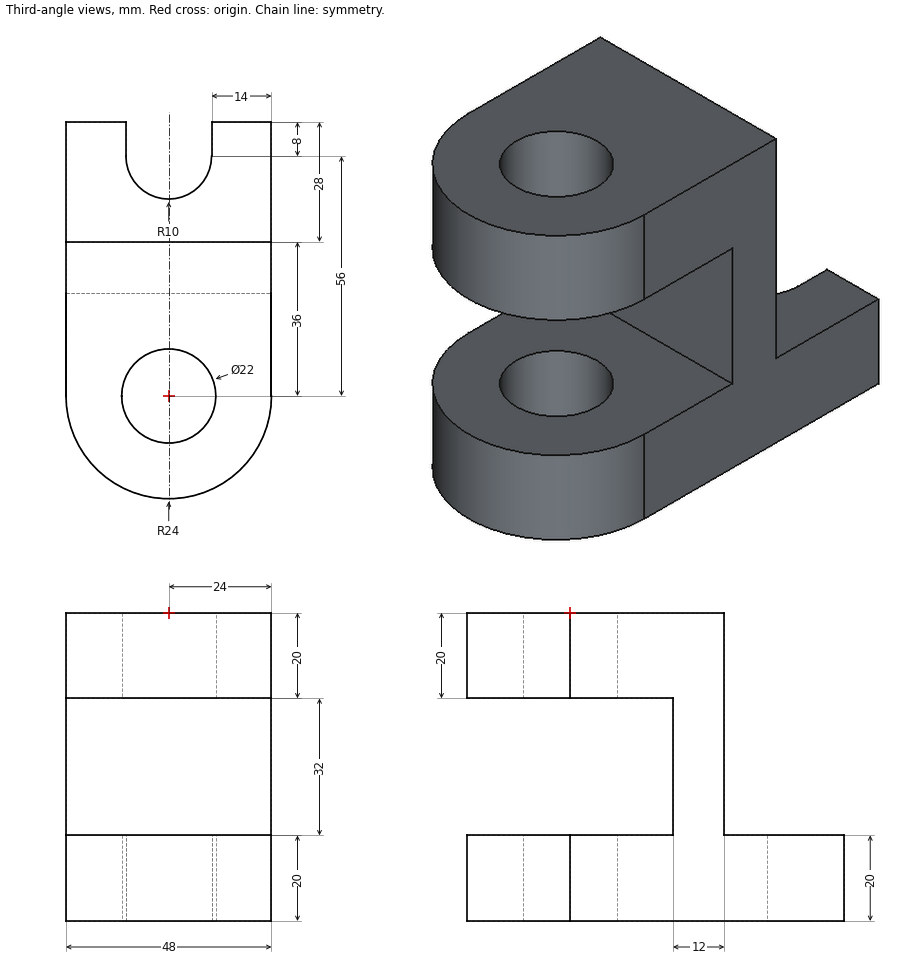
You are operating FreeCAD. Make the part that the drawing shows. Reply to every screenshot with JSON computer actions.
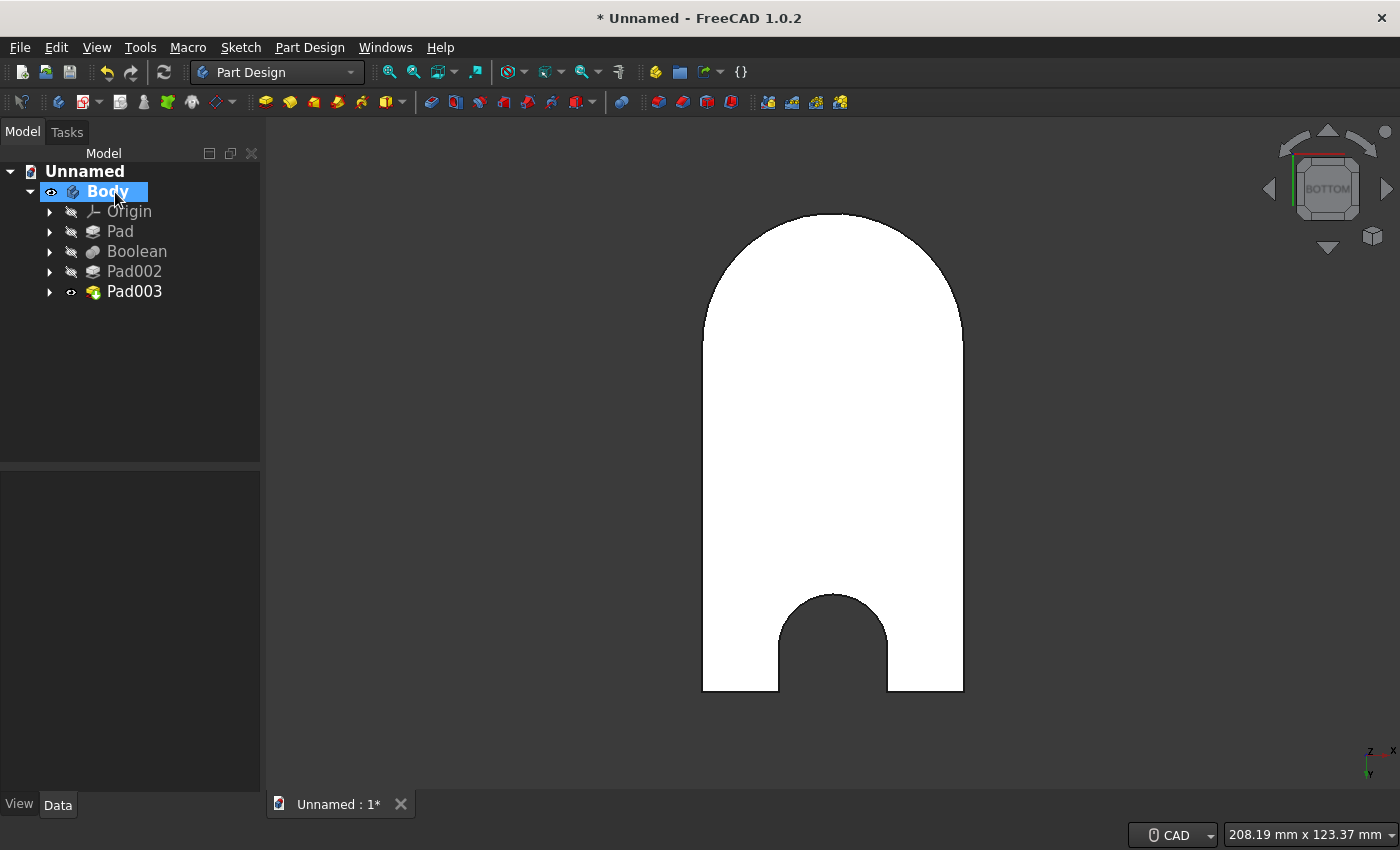
{"action": "key", "text": "0"}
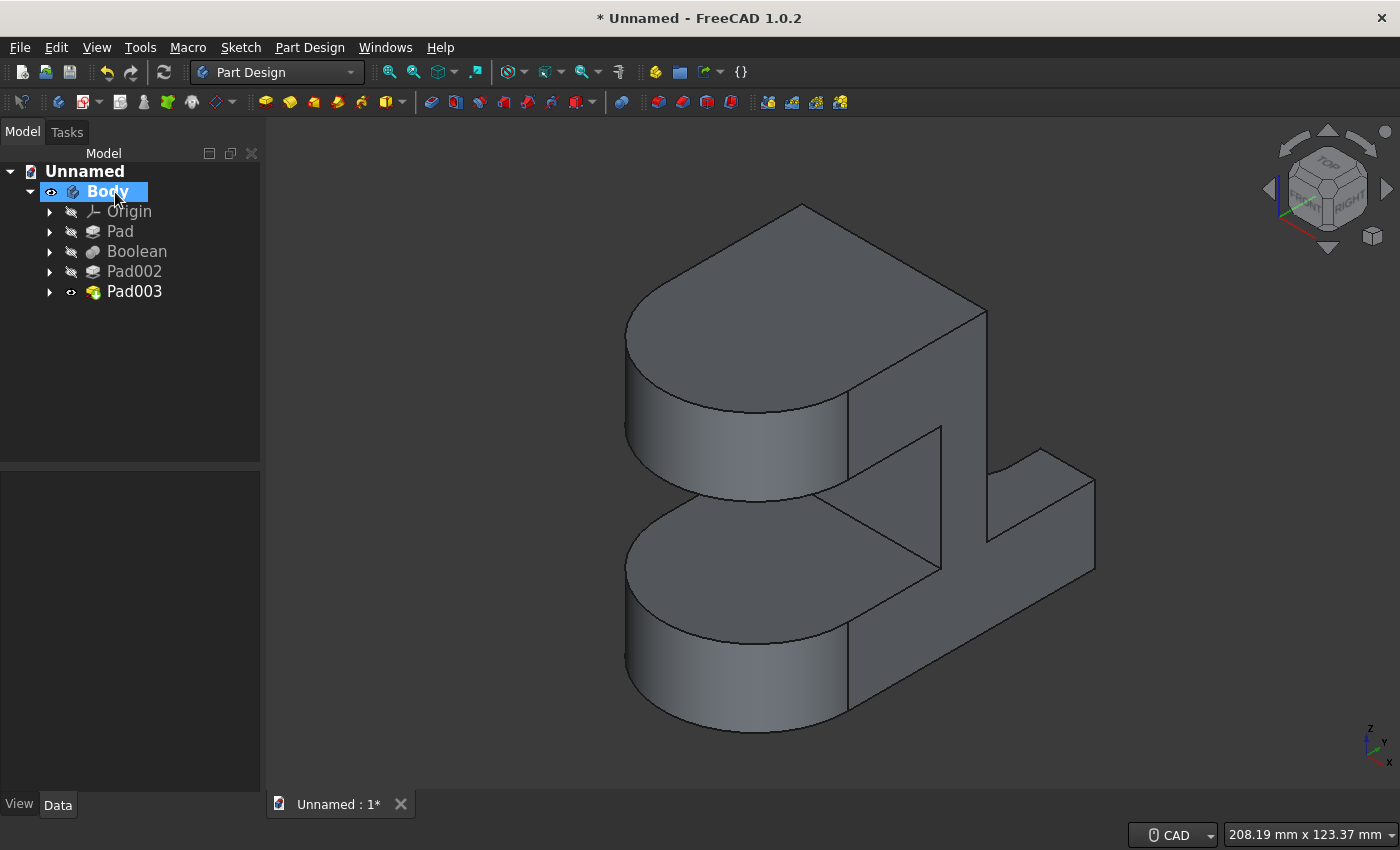
{"action": "left_click", "coordinate": [779, 323]}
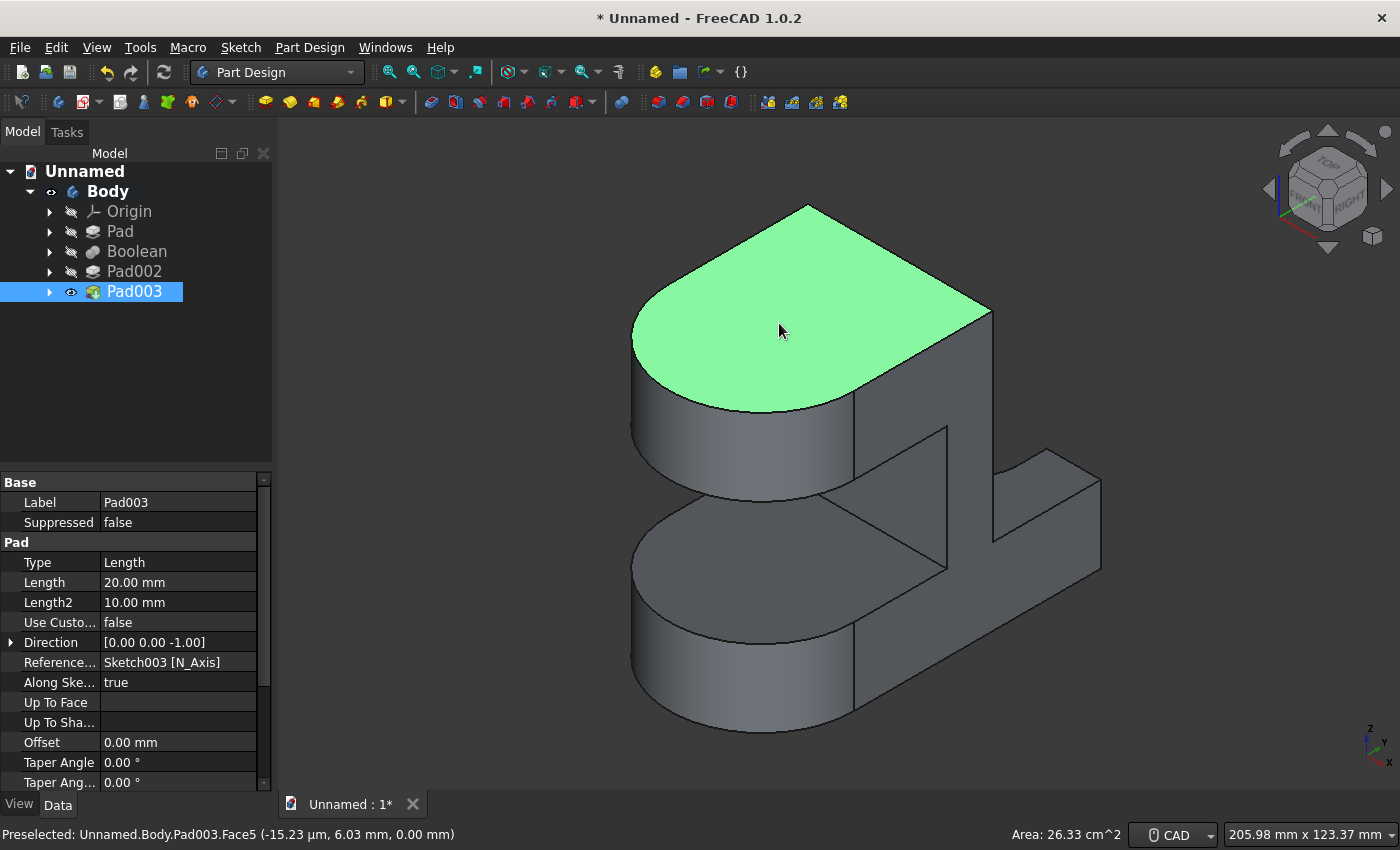
{"action": "left_click", "coordinate": [84, 102]}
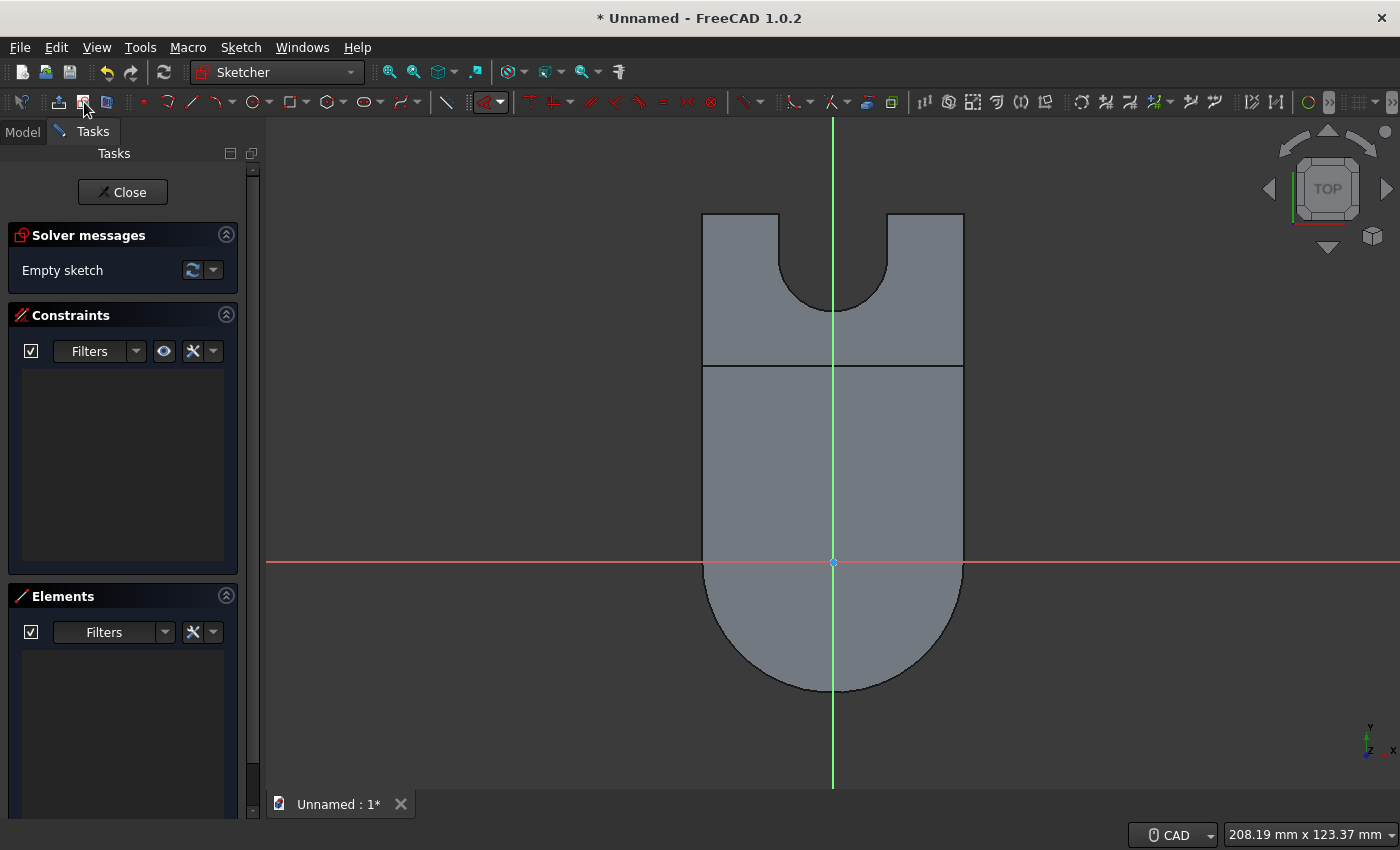
{"action": "scroll", "coordinate": [863, 609], "scroll_direction": "up", "scroll_amount": 6}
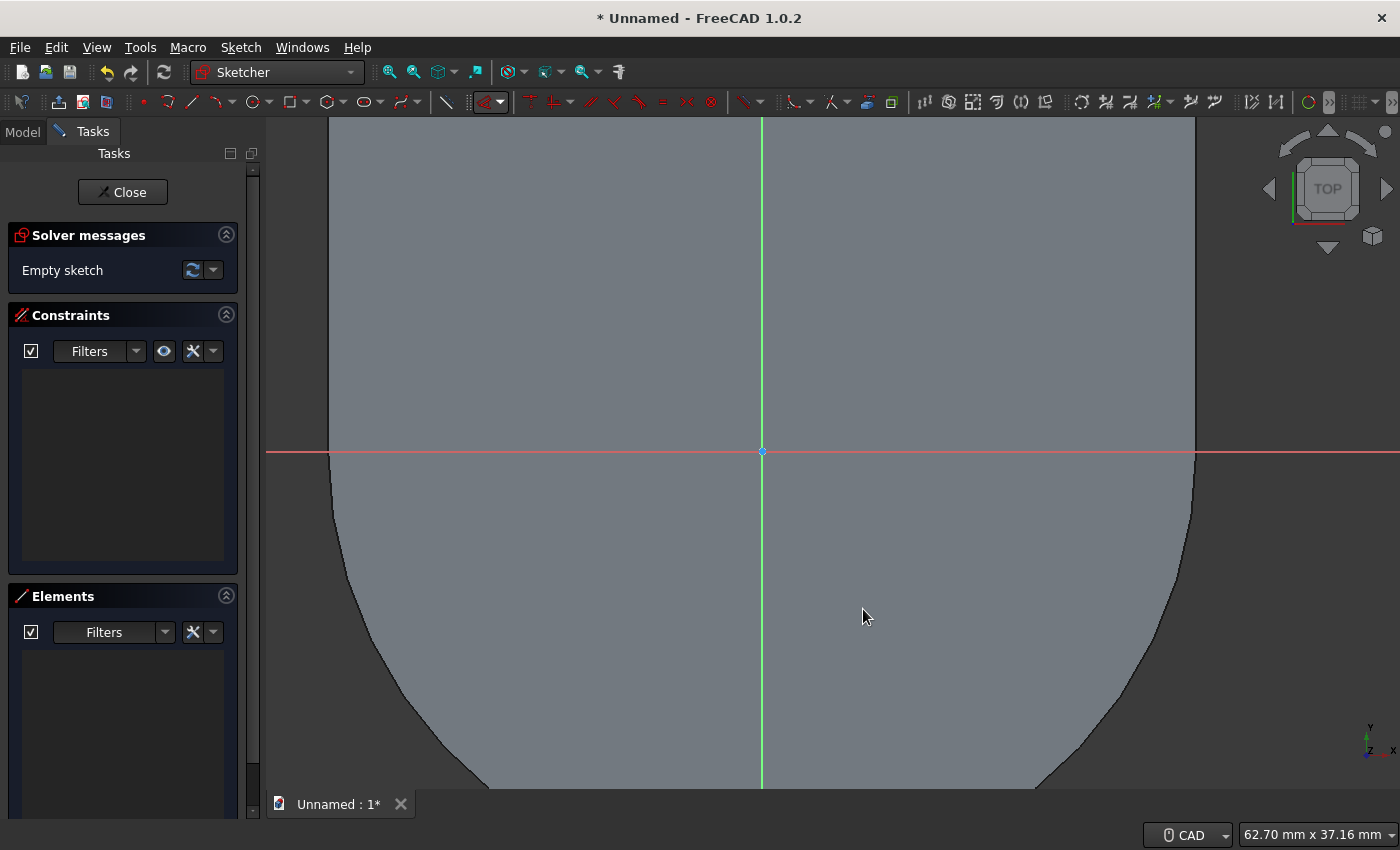
{"action": "left_click", "coordinate": [254, 102]}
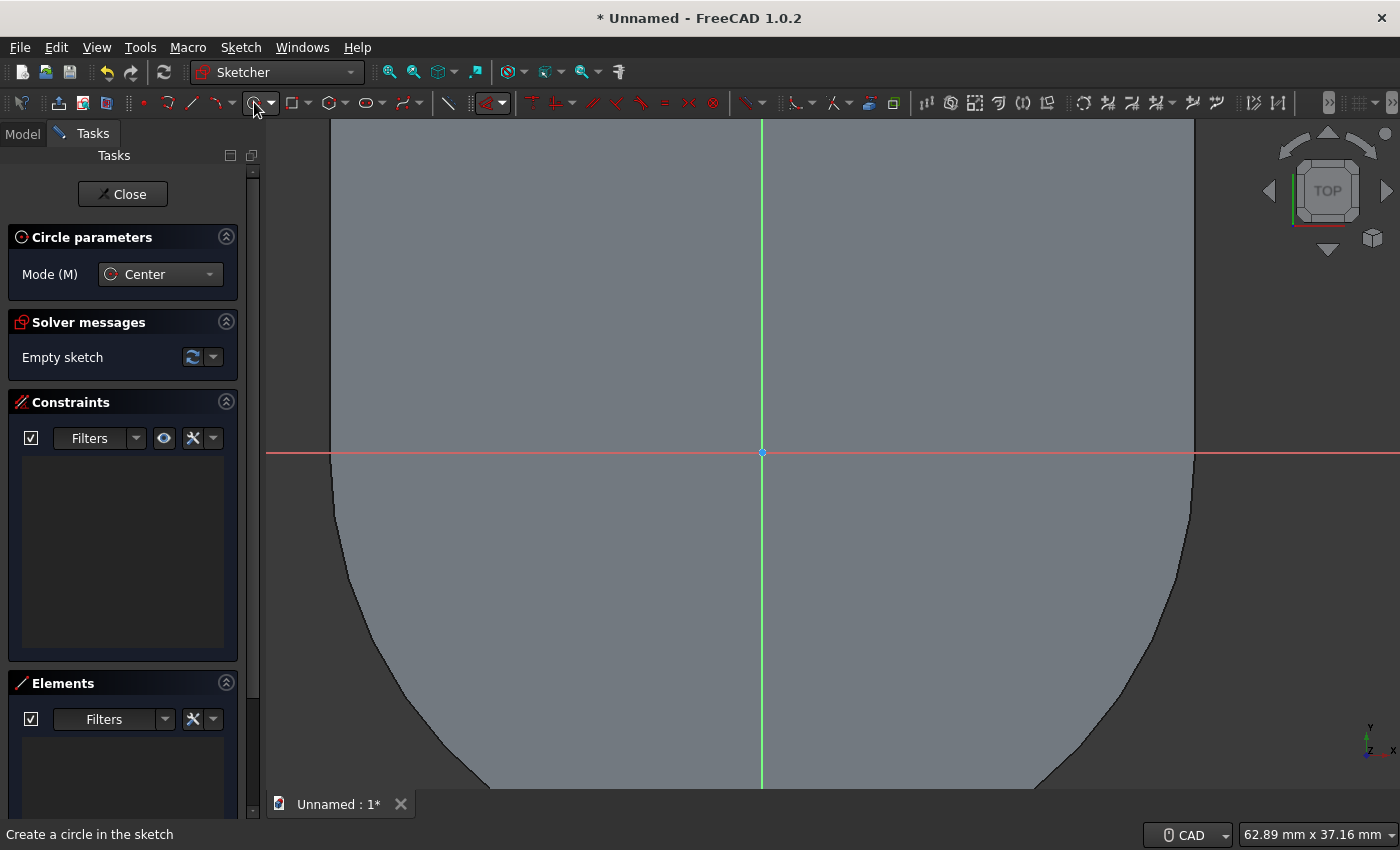
{"action": "left_click", "coordinate": [762, 453]}
{"action": "left_click", "coordinate": [903, 312]}
{"action": "key", "text": "Escape"}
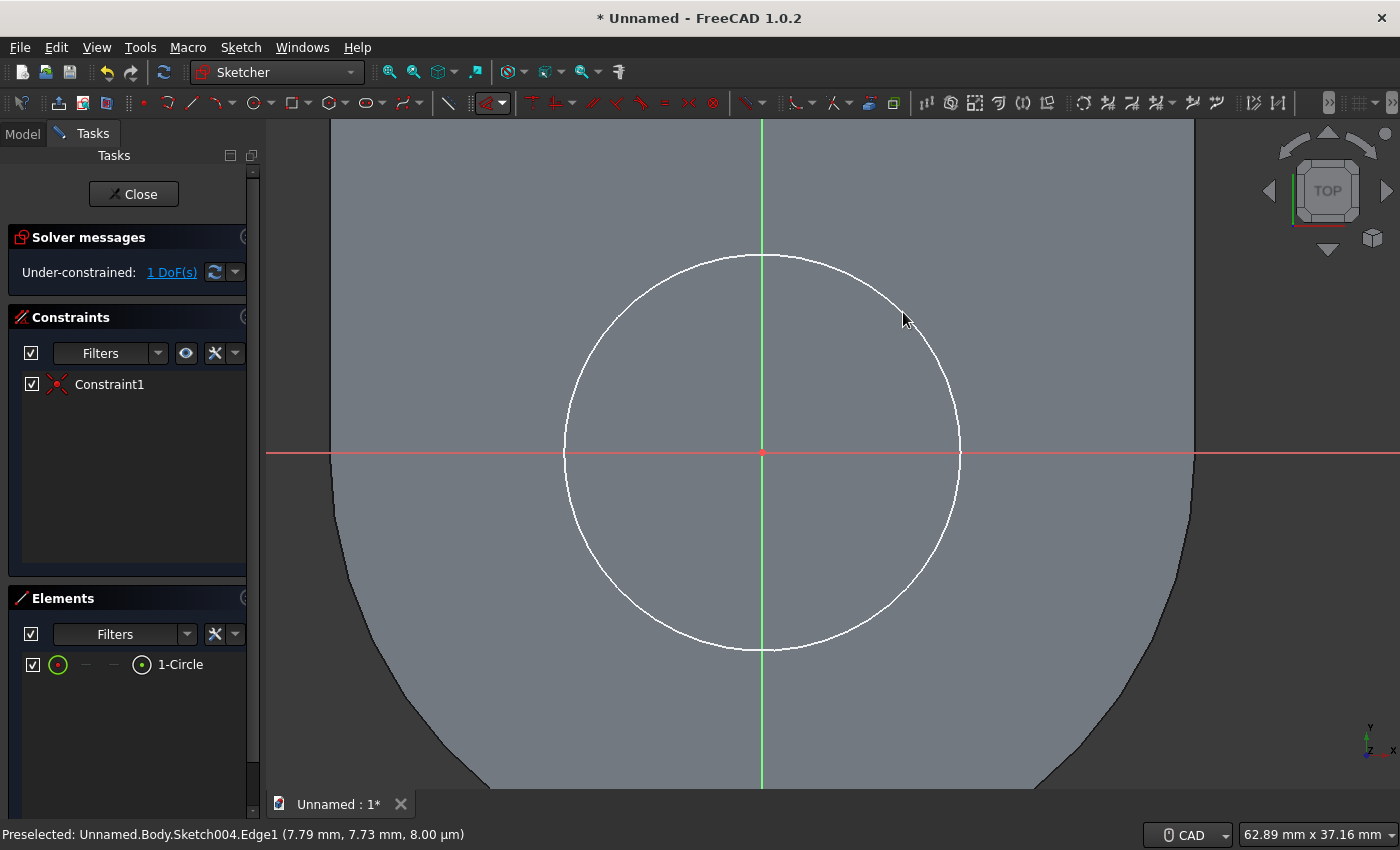
{"action": "left_click", "coordinate": [902, 312]}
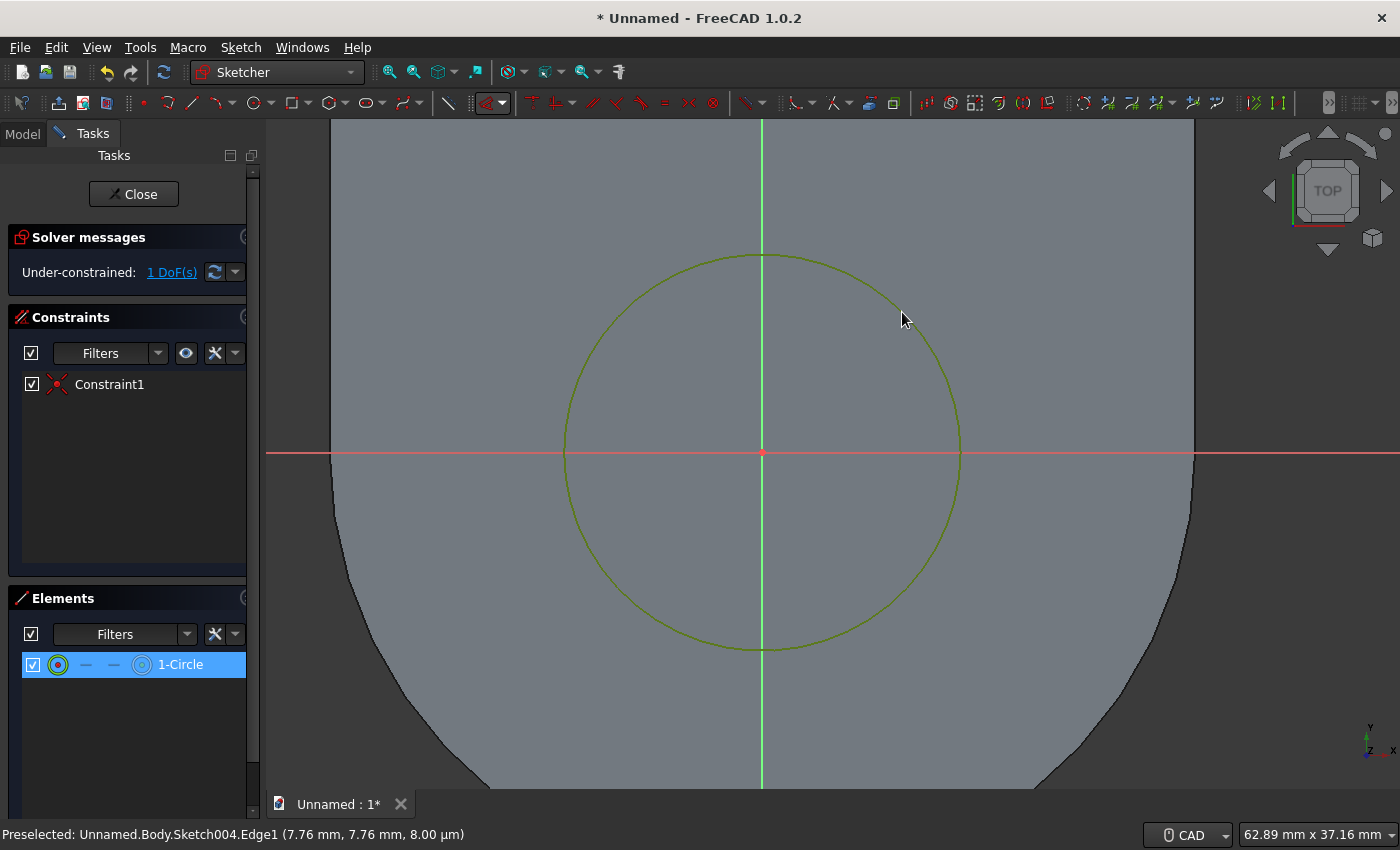
{"action": "key", "text": "k o"}